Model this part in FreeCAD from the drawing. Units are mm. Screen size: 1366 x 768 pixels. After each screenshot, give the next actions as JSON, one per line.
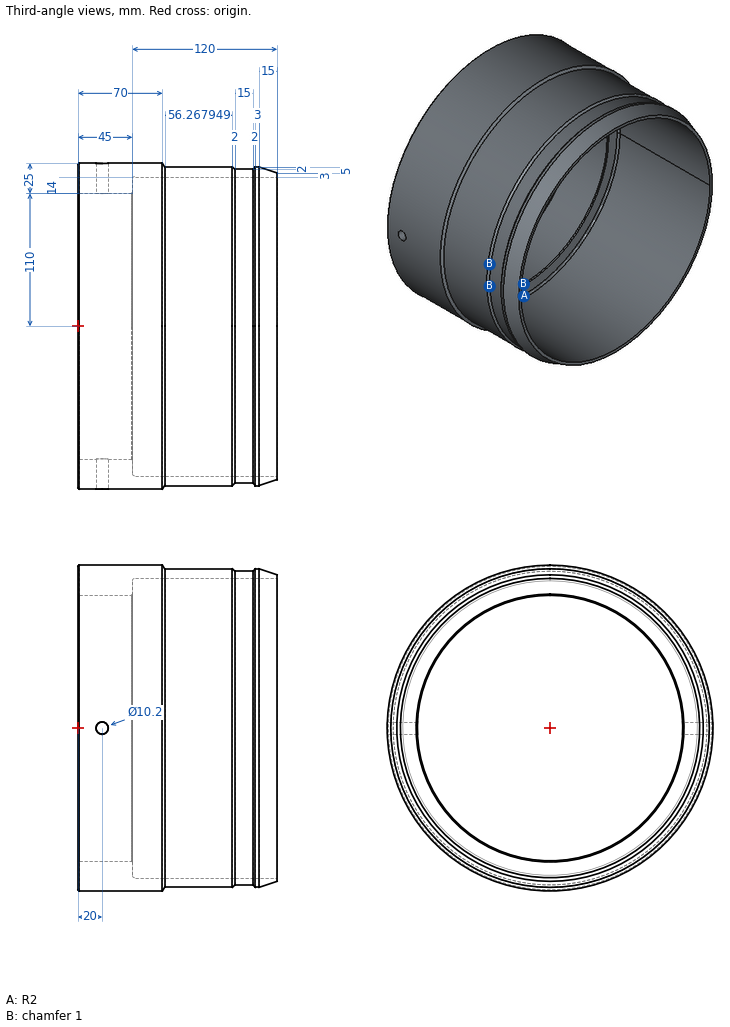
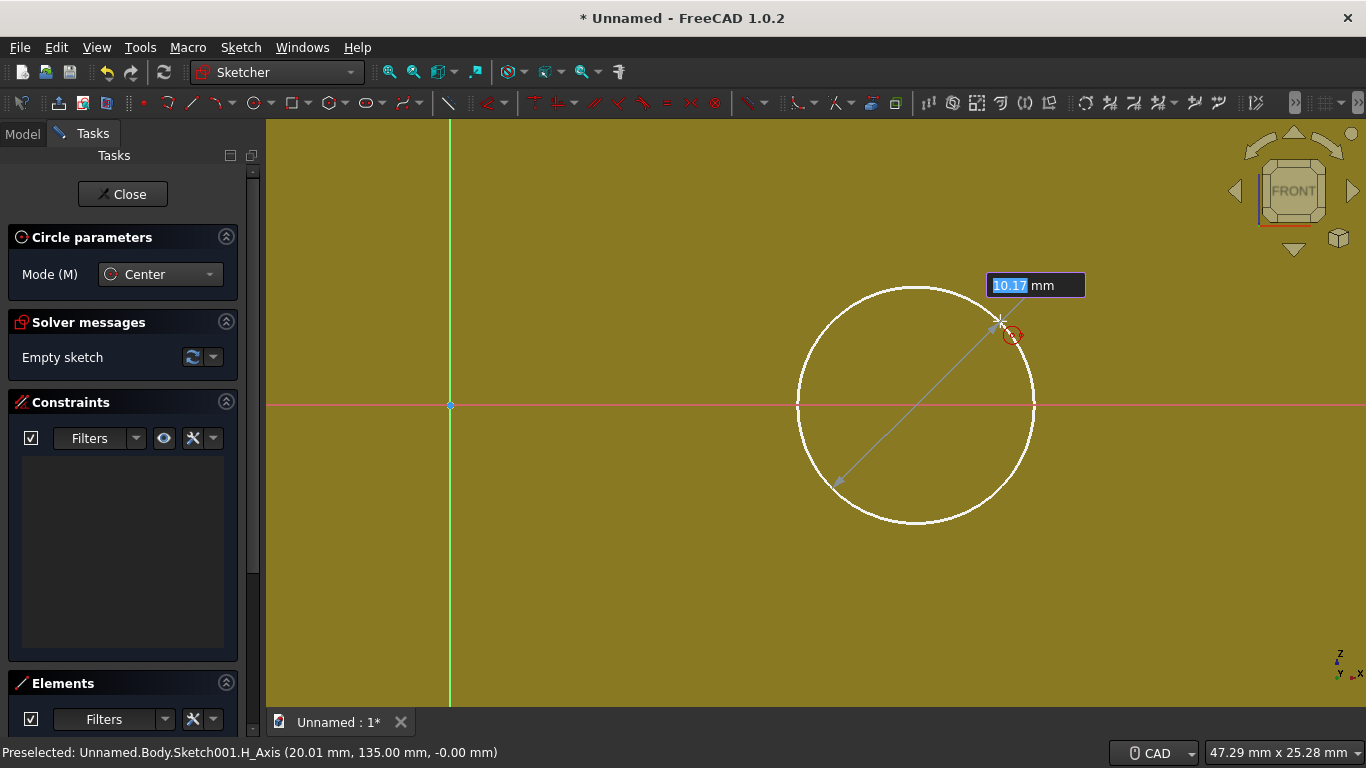
{"action": "type", "text": "10.2"}
{"action": "key", "text": "Return"}
{"action": "key", "text": "Escape"}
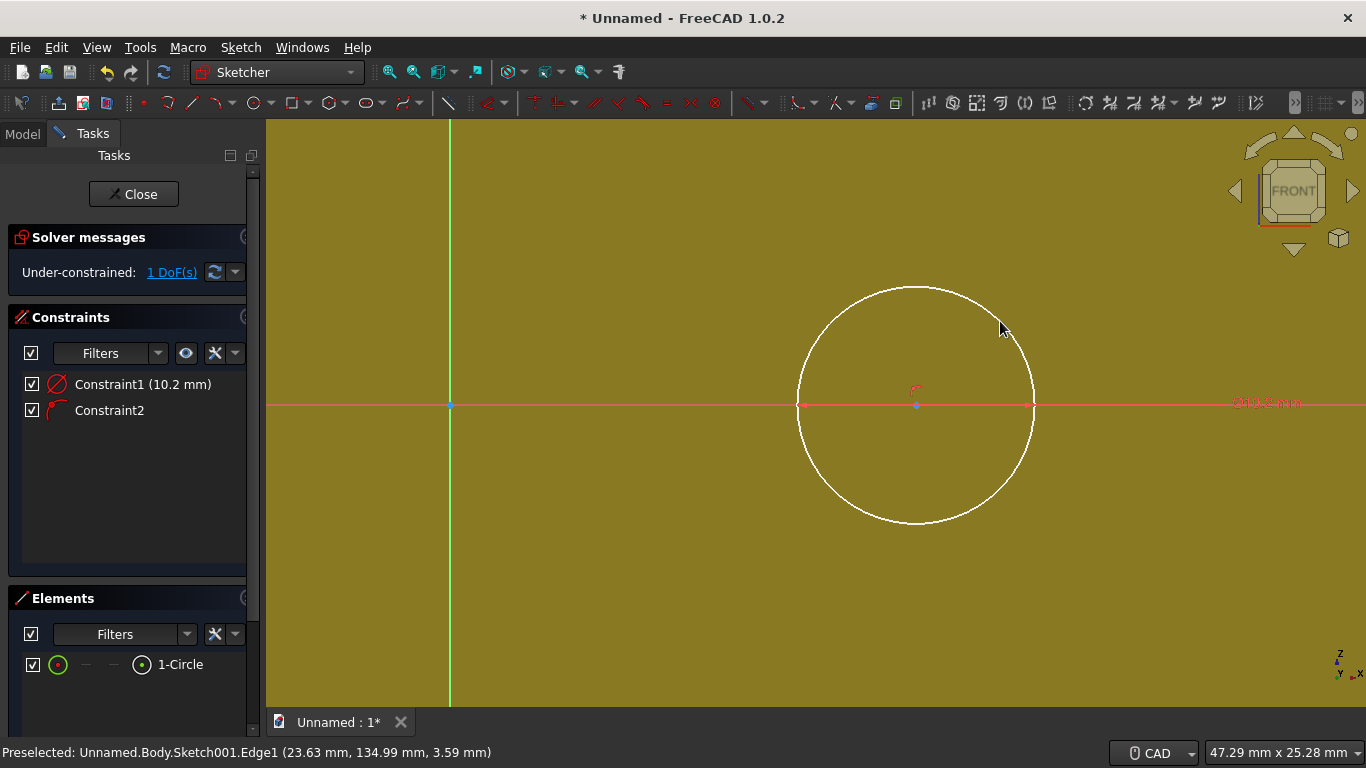
{"action": "left_click", "coordinate": [488, 104]}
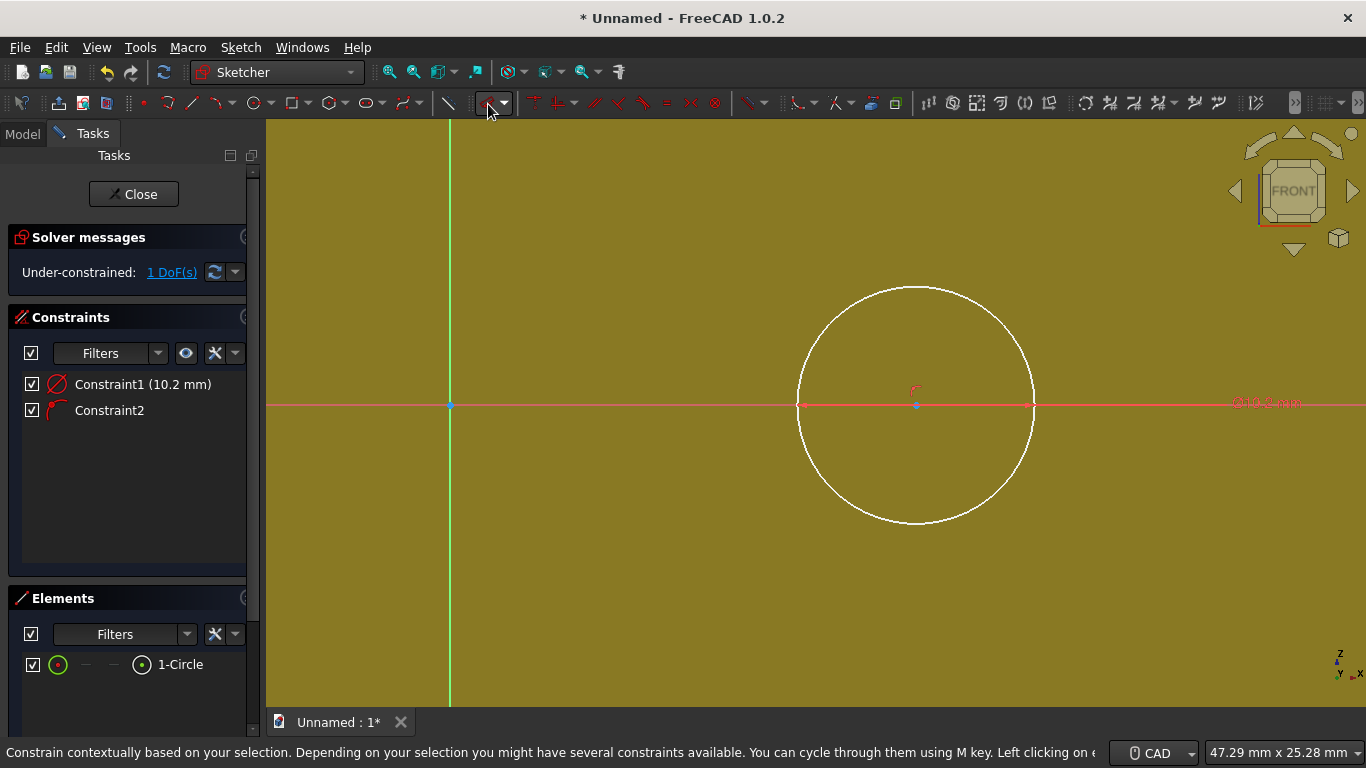
{"action": "left_click", "coordinate": [916, 405]}
{"action": "left_click", "coordinate": [683, 439]}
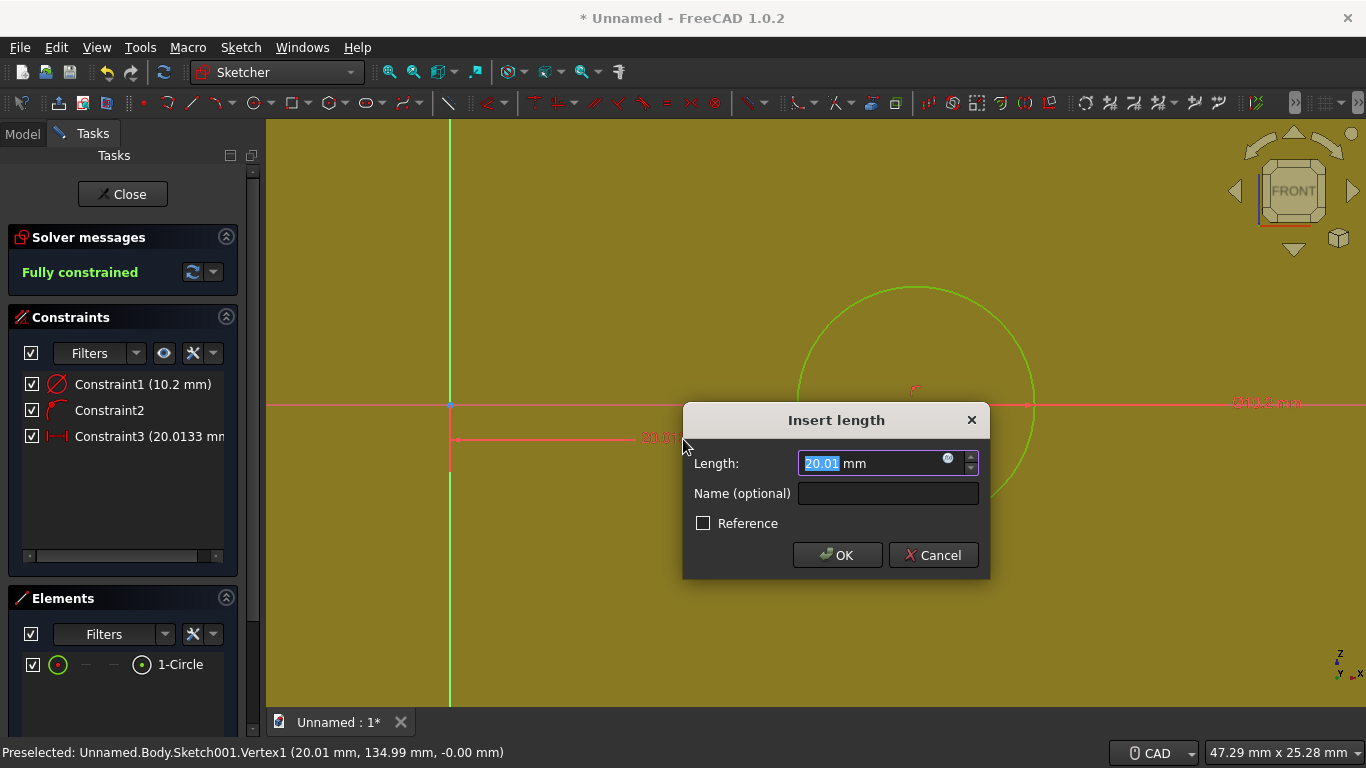
{"action": "type", "text": "20"}
{"action": "key", "text": "Return"}
{"action": "key", "text": "Escape"}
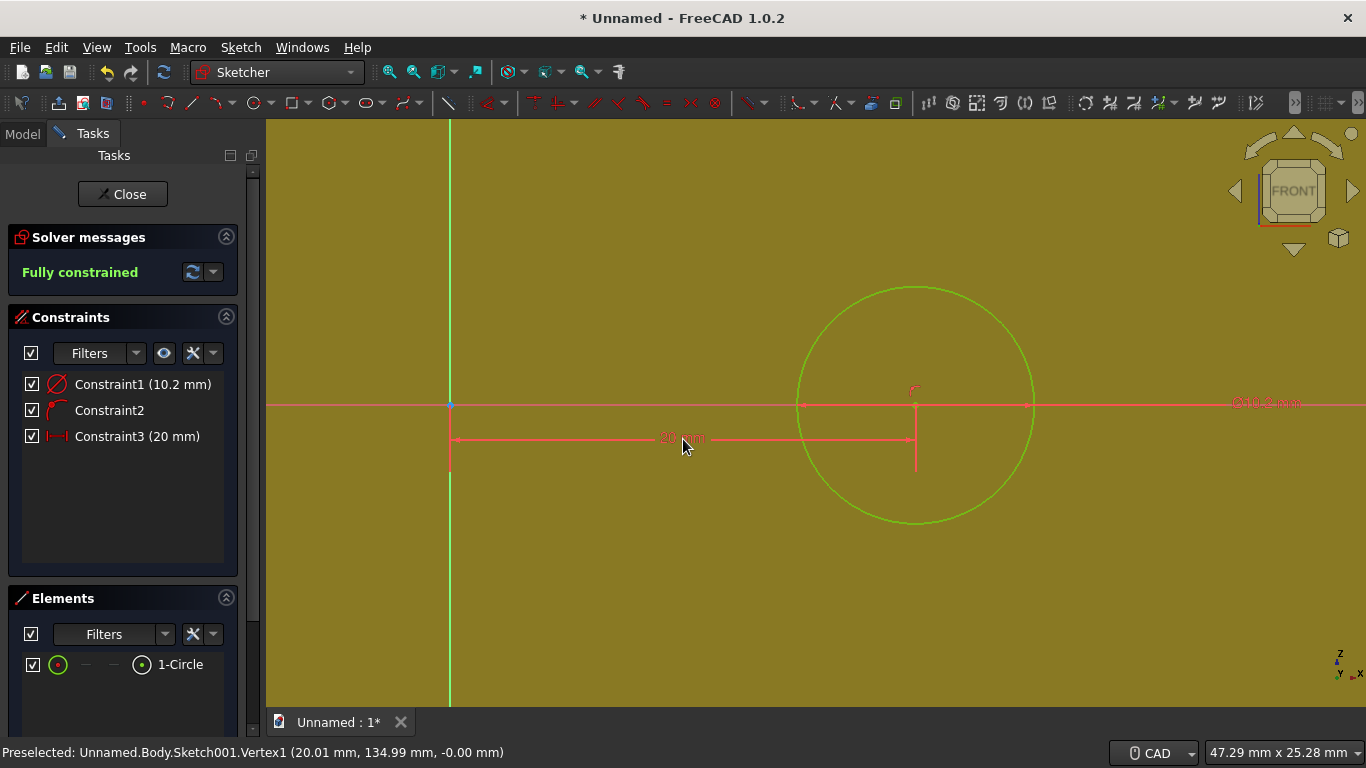
{"action": "left_click", "coordinate": [123, 194]}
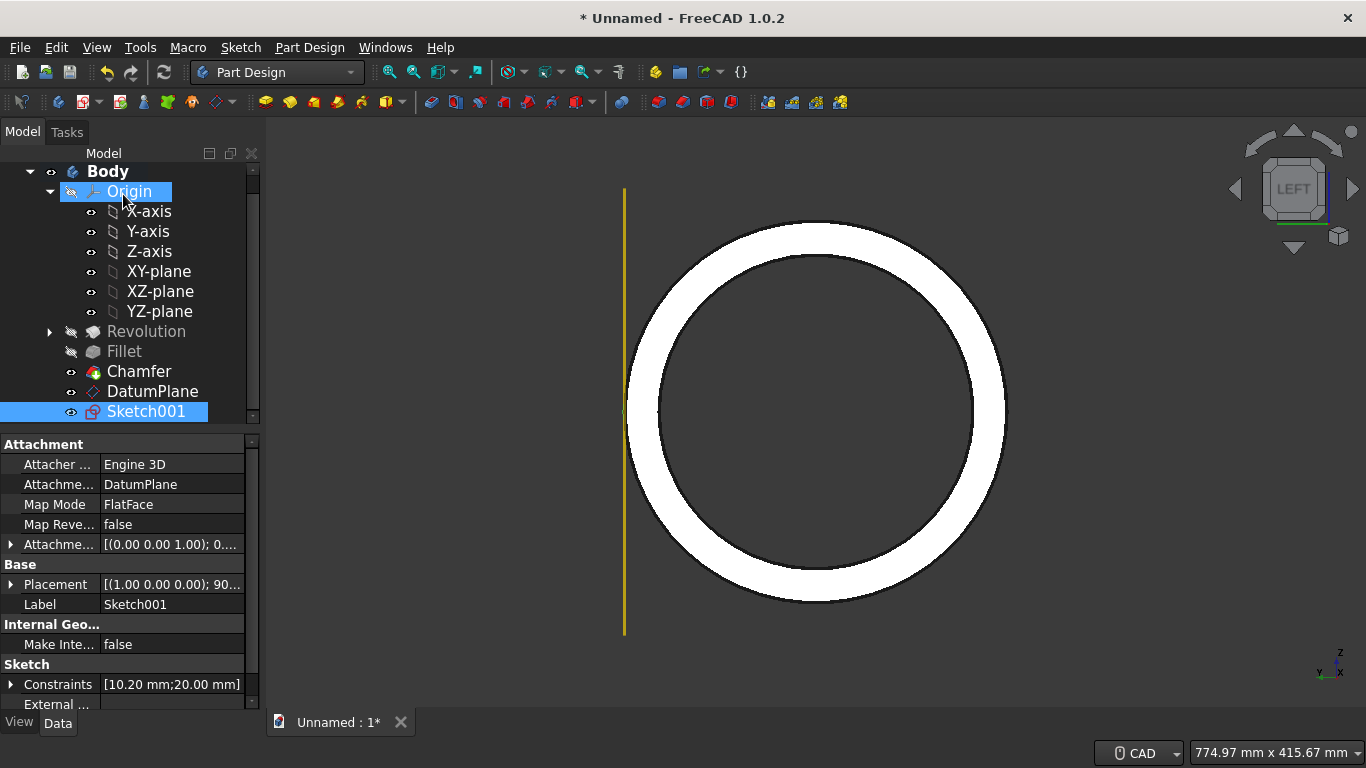
{"action": "left_click", "coordinate": [432, 102]}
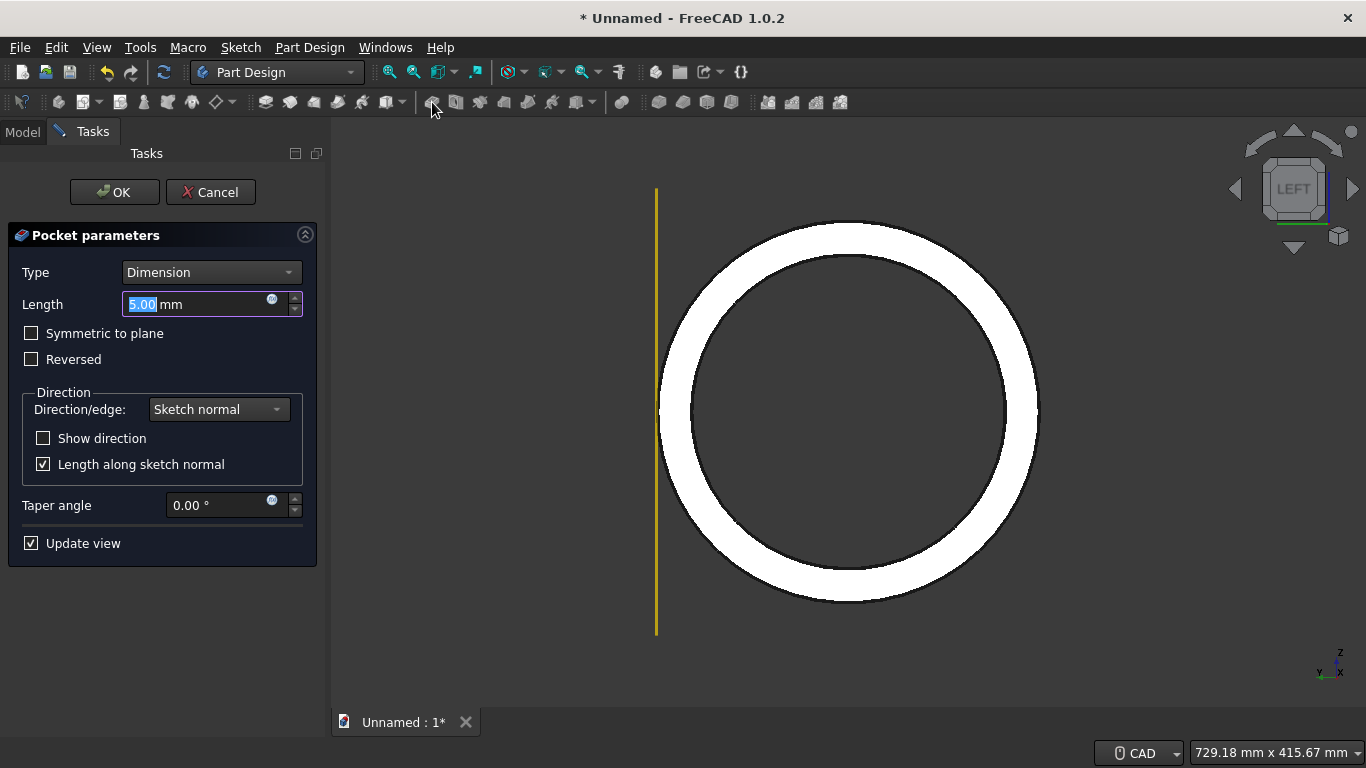
{"action": "left_click", "coordinate": [212, 272]}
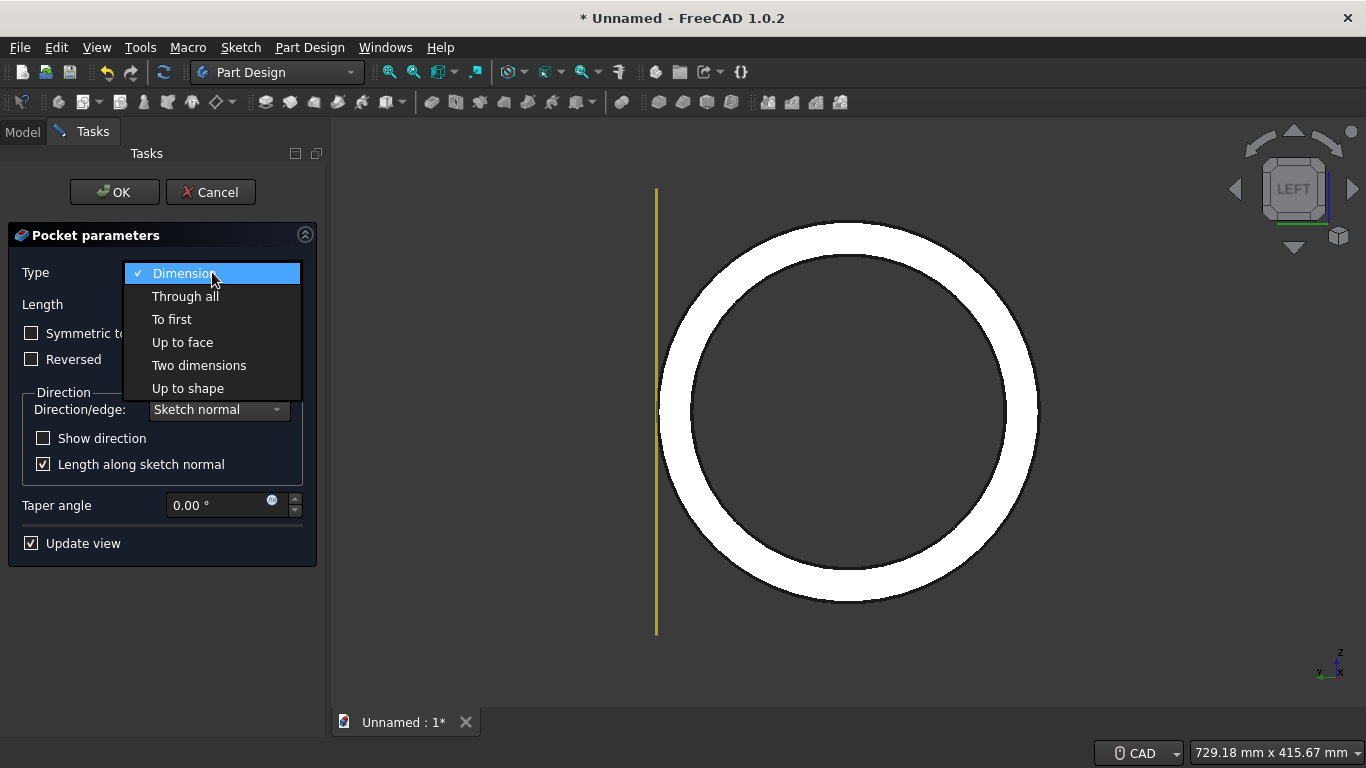
{"action": "left_click", "coordinate": [212, 296]}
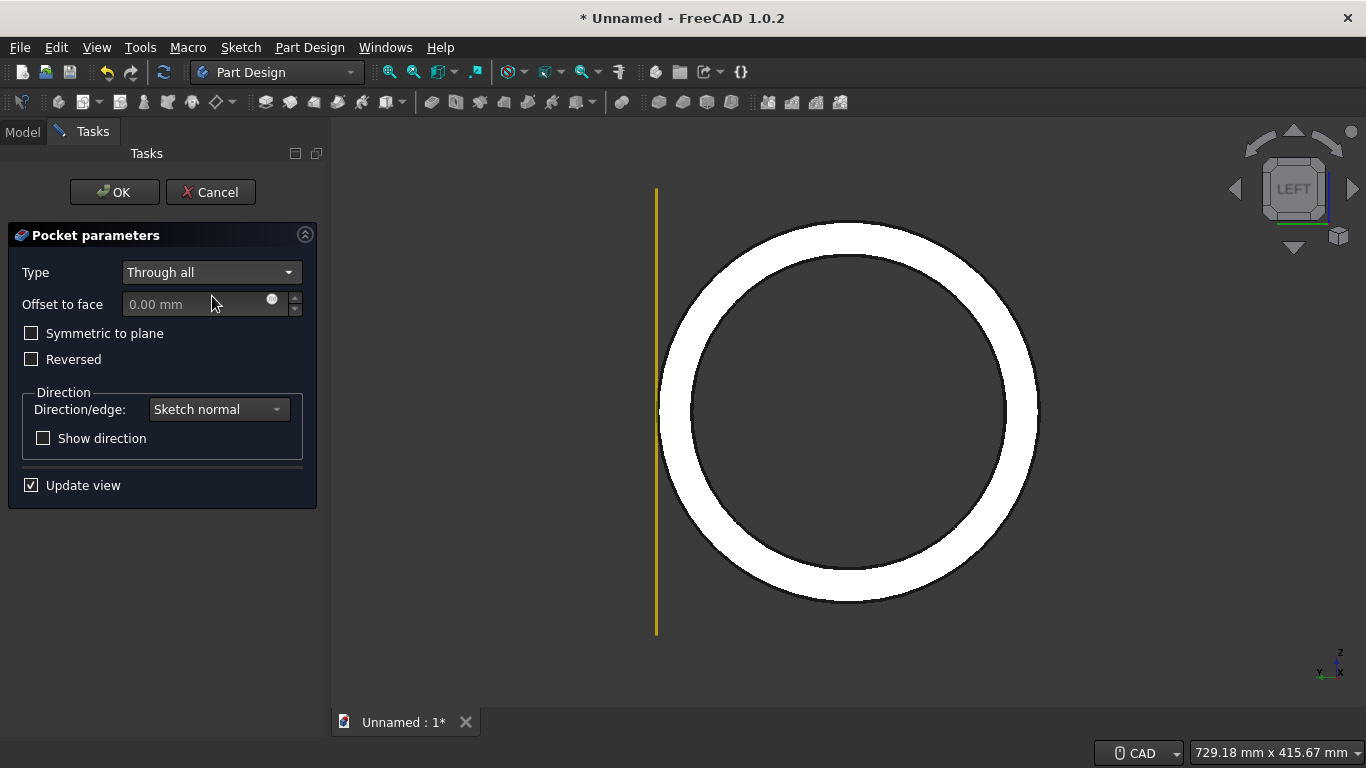
{"action": "left_click", "coordinate": [30, 359]}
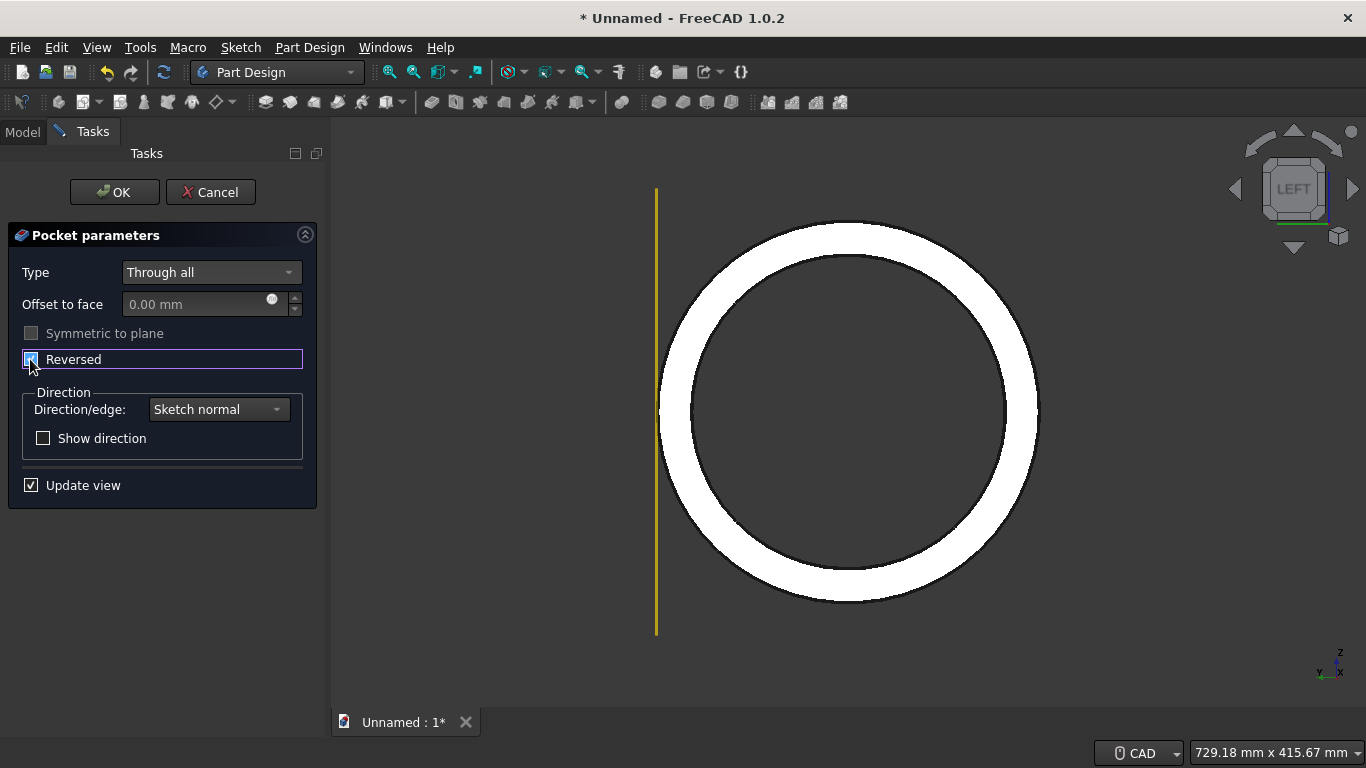
{"action": "left_click", "coordinate": [115, 192]}